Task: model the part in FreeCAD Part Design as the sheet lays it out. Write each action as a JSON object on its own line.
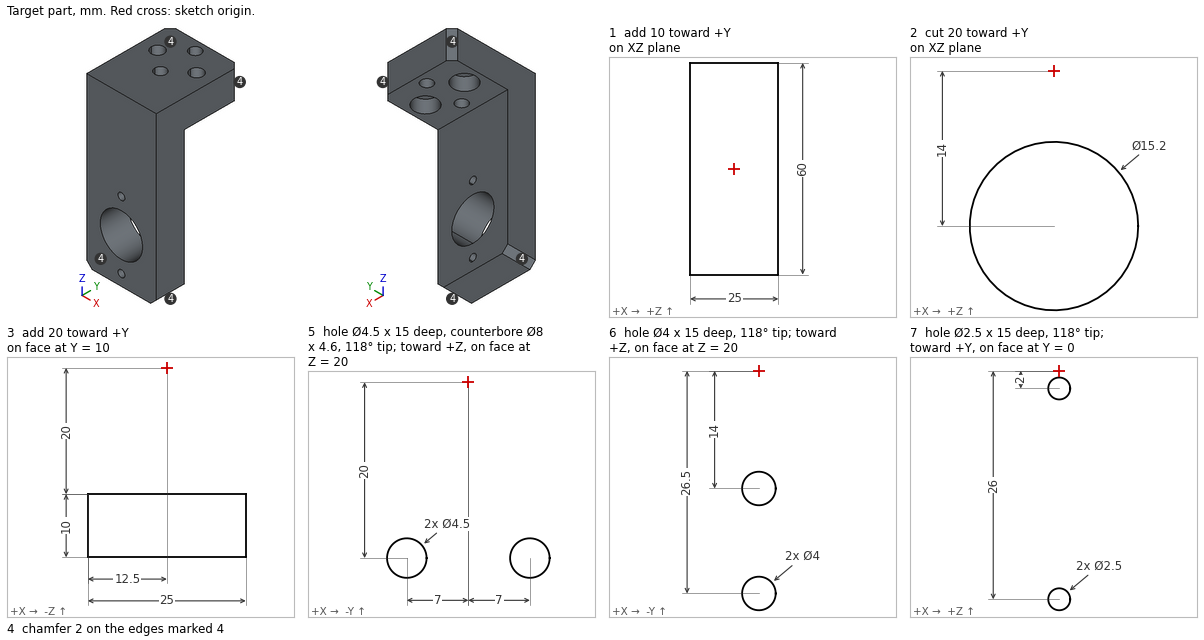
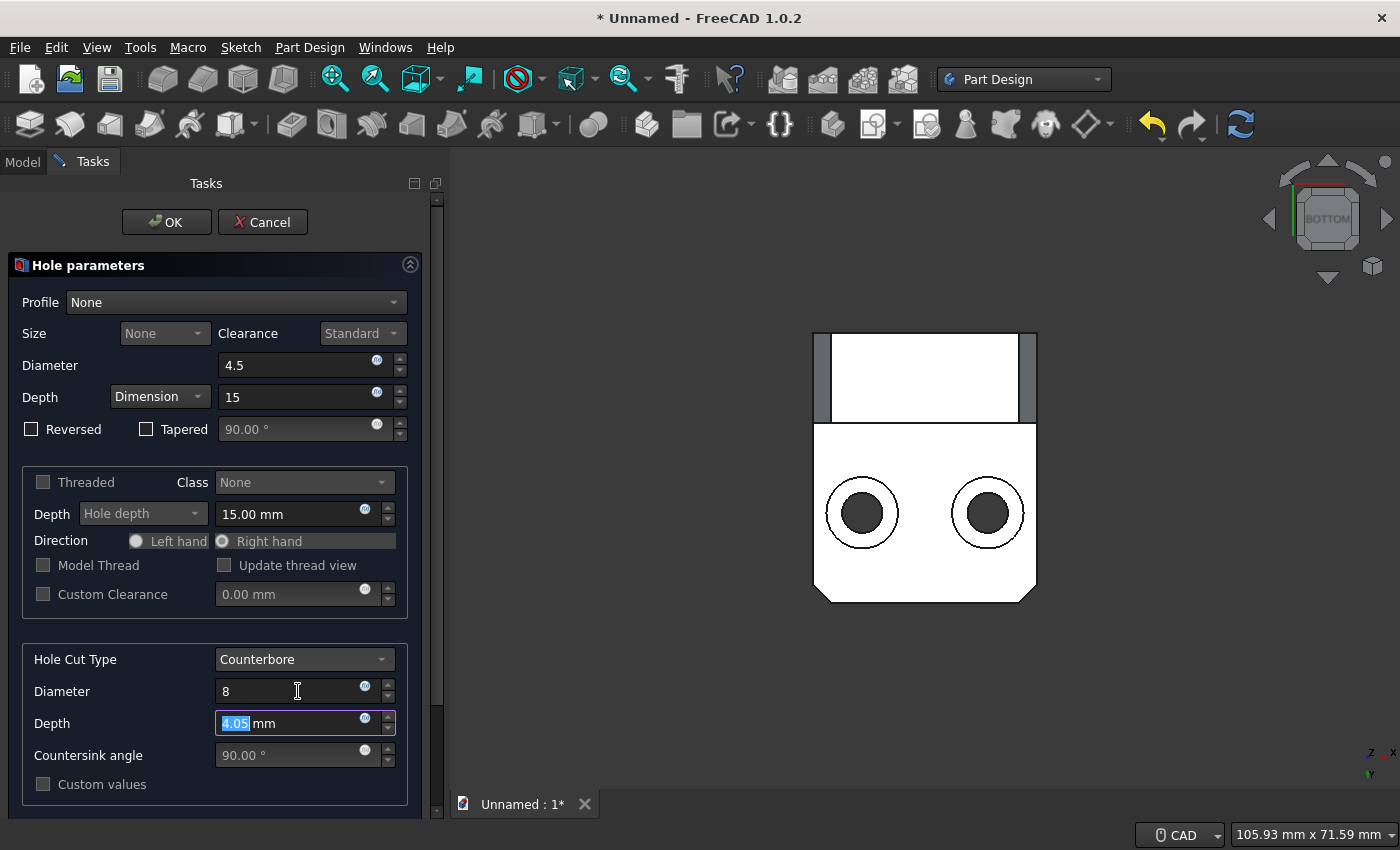
{"action": "type", "text": "4.6"}
{"action": "key", "text": "Tab"}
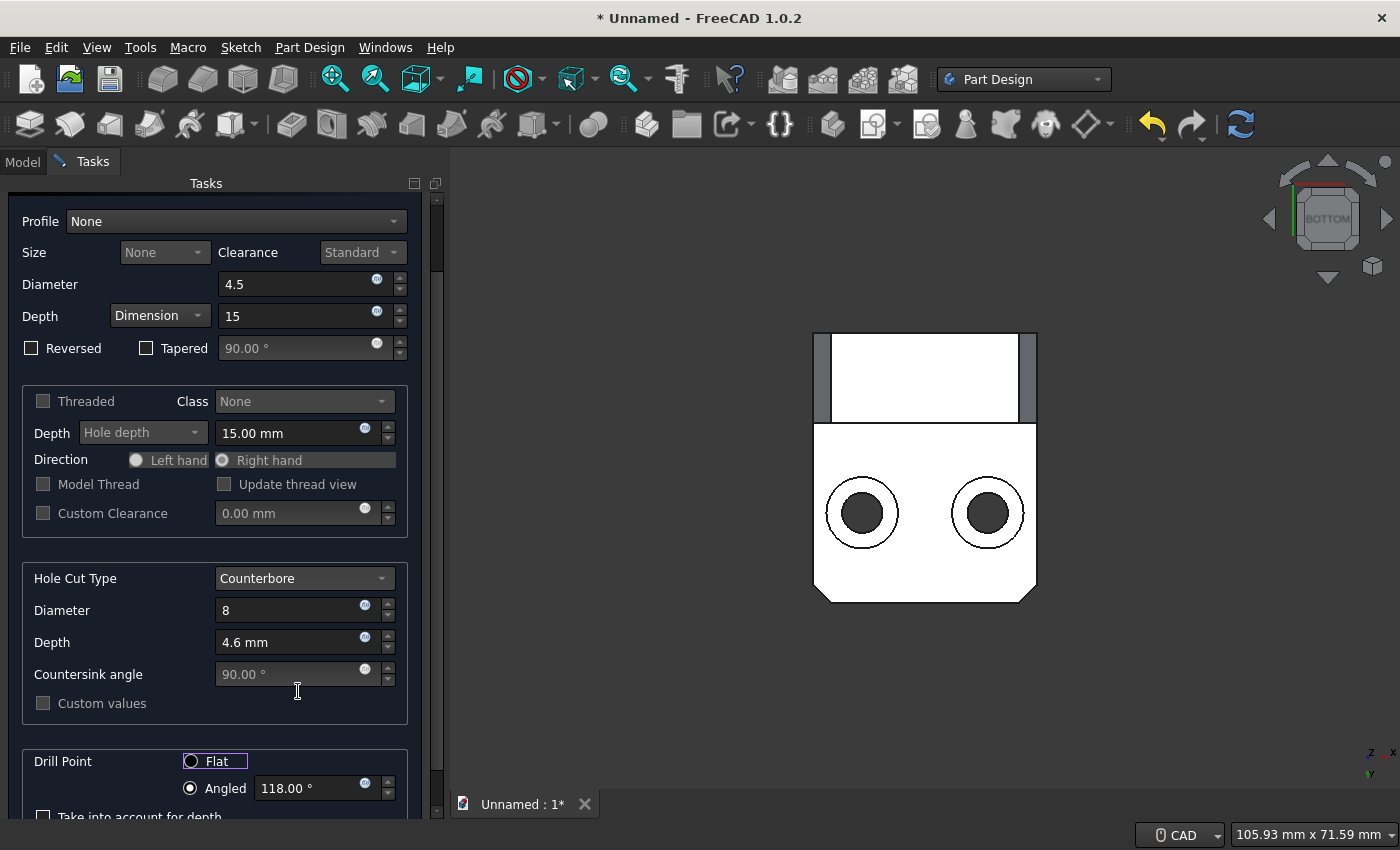
{"action": "scroll", "coordinate": [437, 506], "scroll_direction": "up", "scroll_amount": 3}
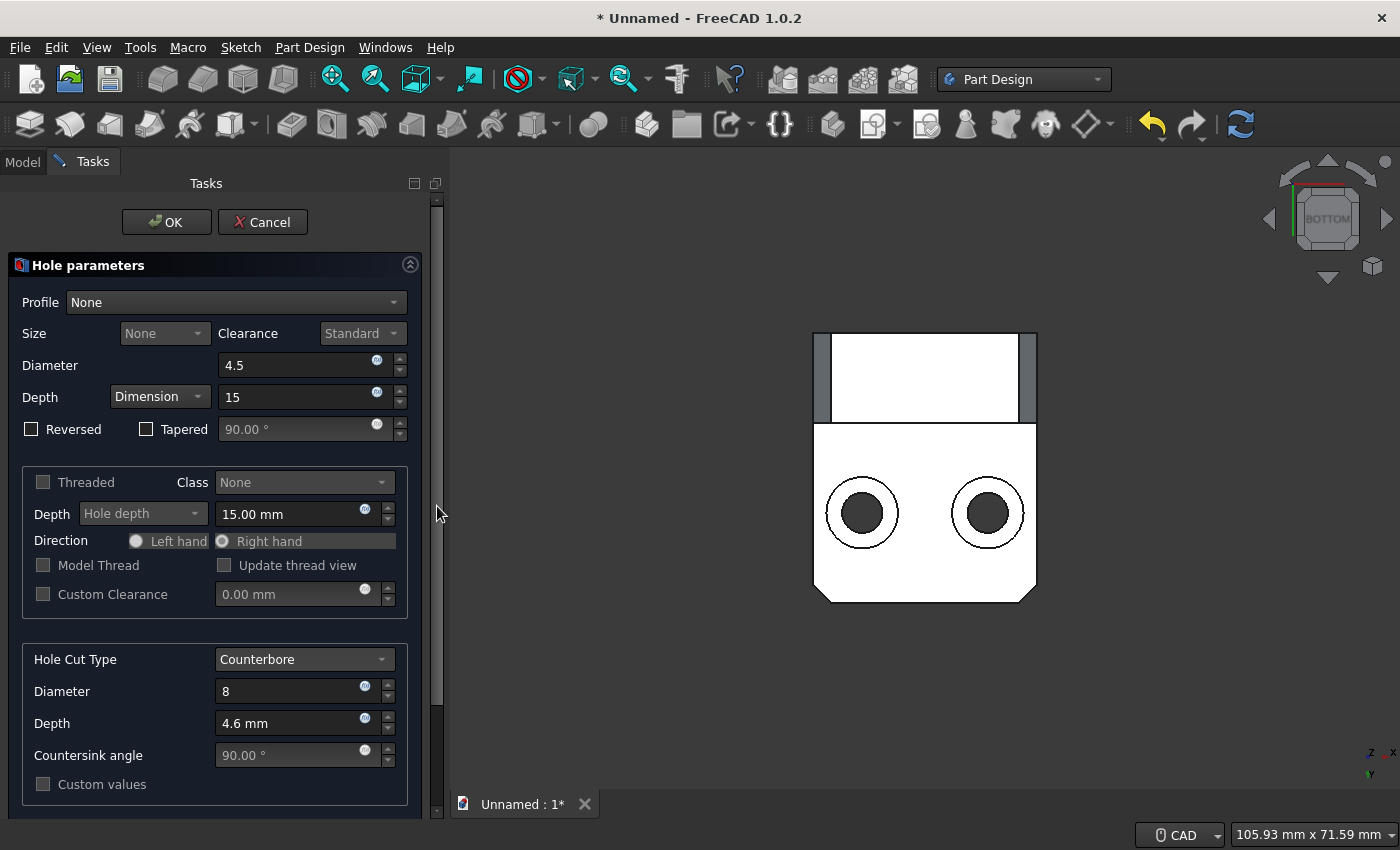
{"action": "left_click", "coordinate": [167, 222]}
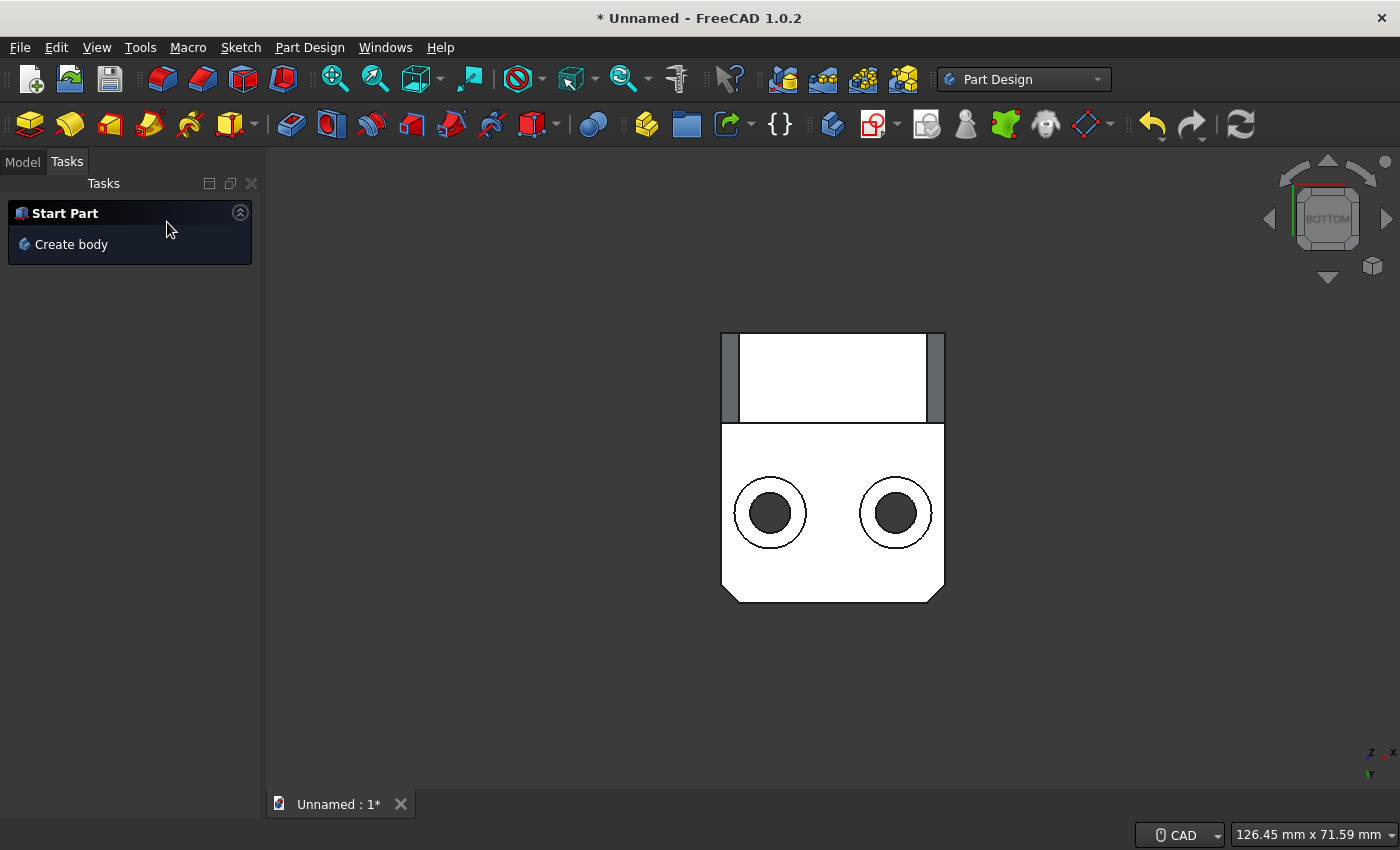
{"action": "key", "text": "v f"}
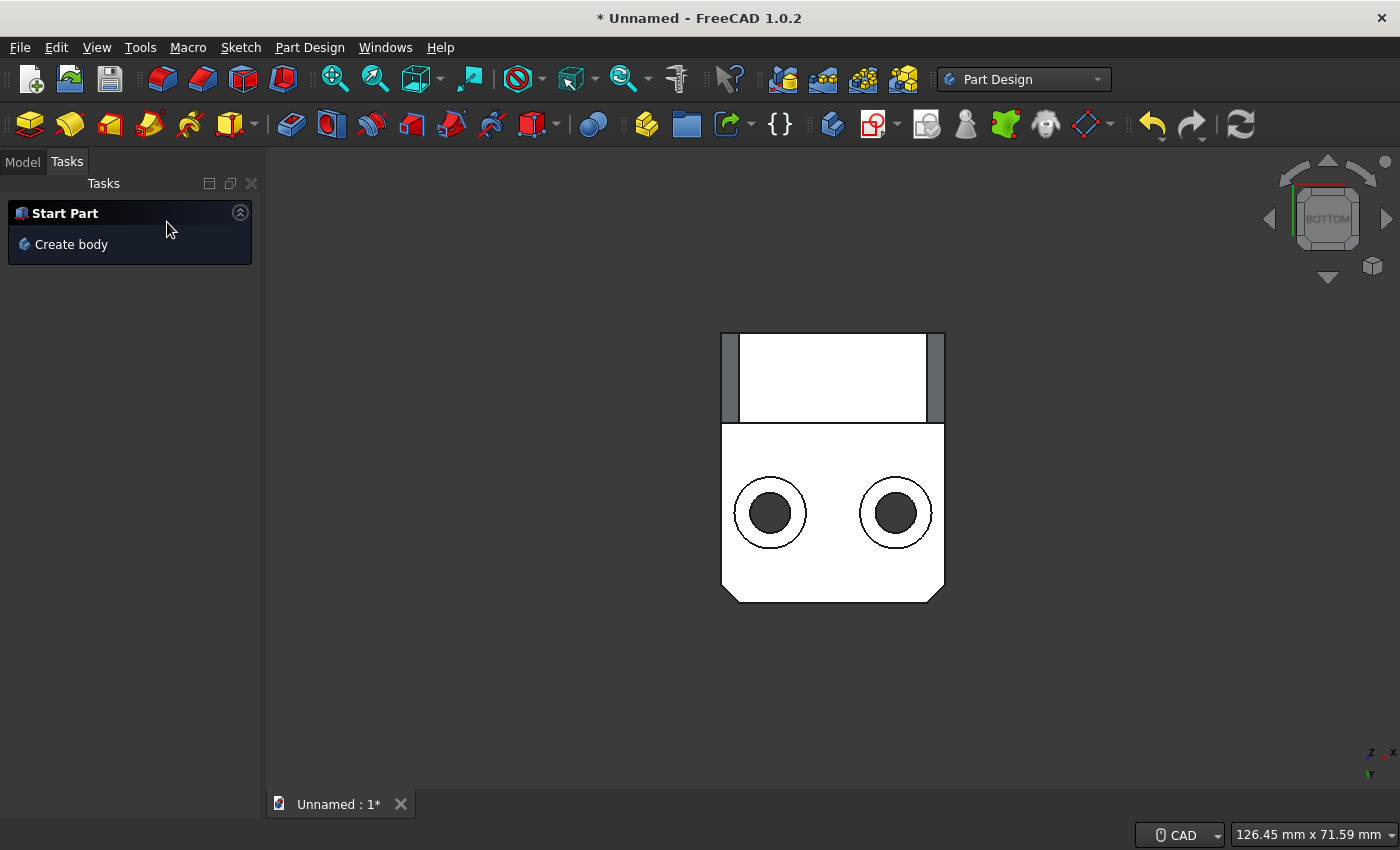
{"action": "left_click", "coordinate": [833, 461]}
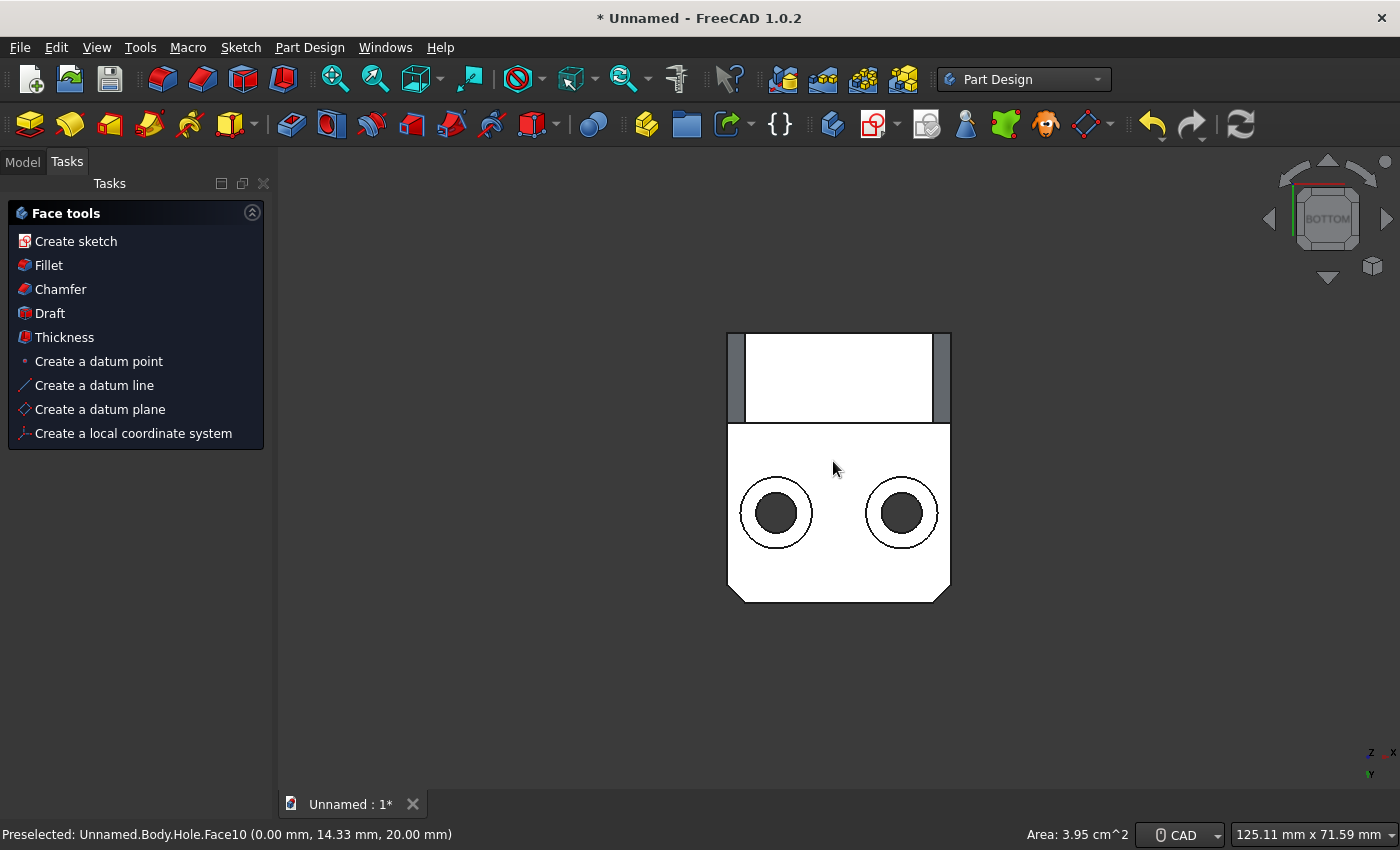
{"action": "left_click", "coordinate": [874, 124]}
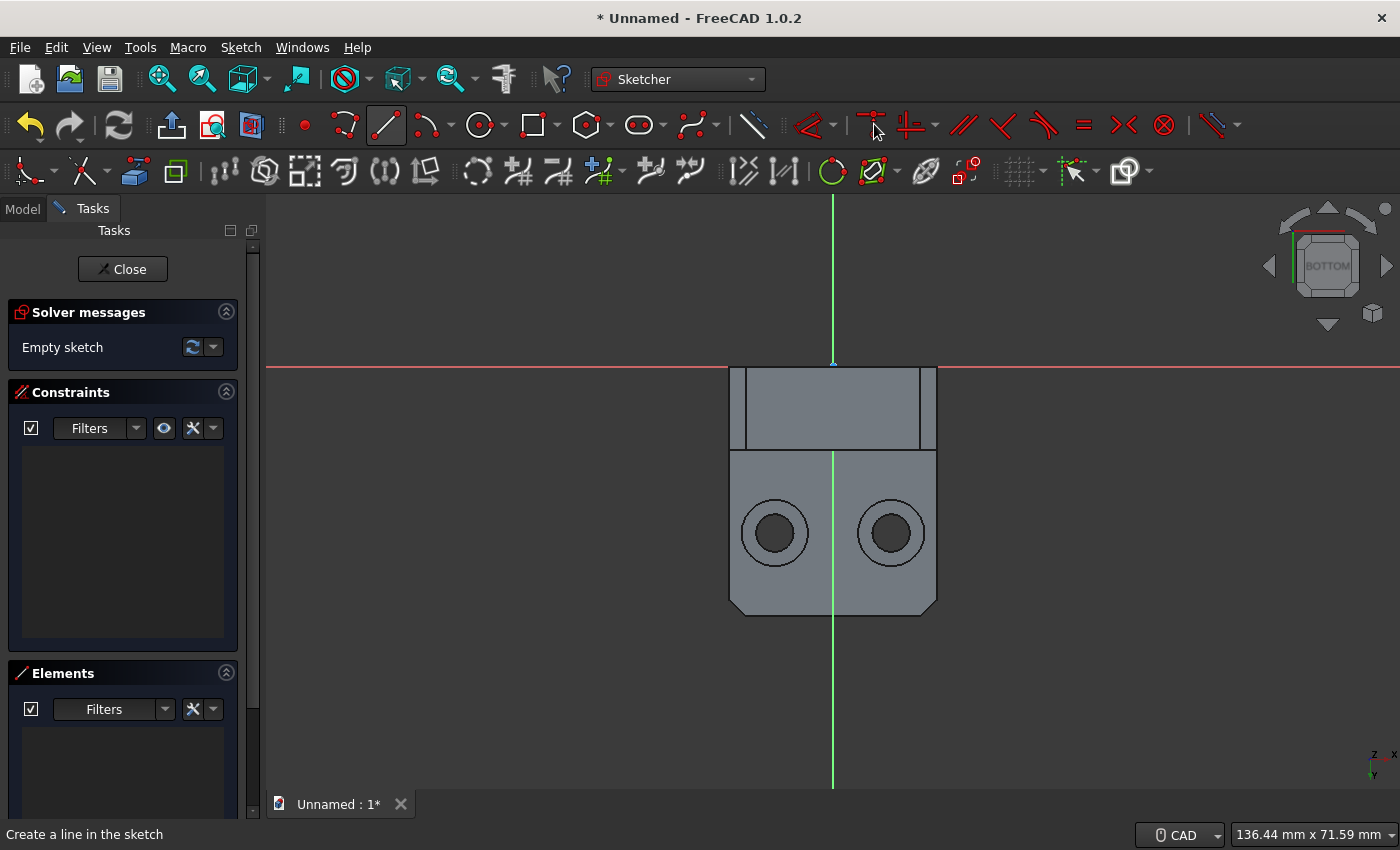
{"action": "scroll", "coordinate": [972, 473], "scroll_direction": "up", "scroll_amount": 2}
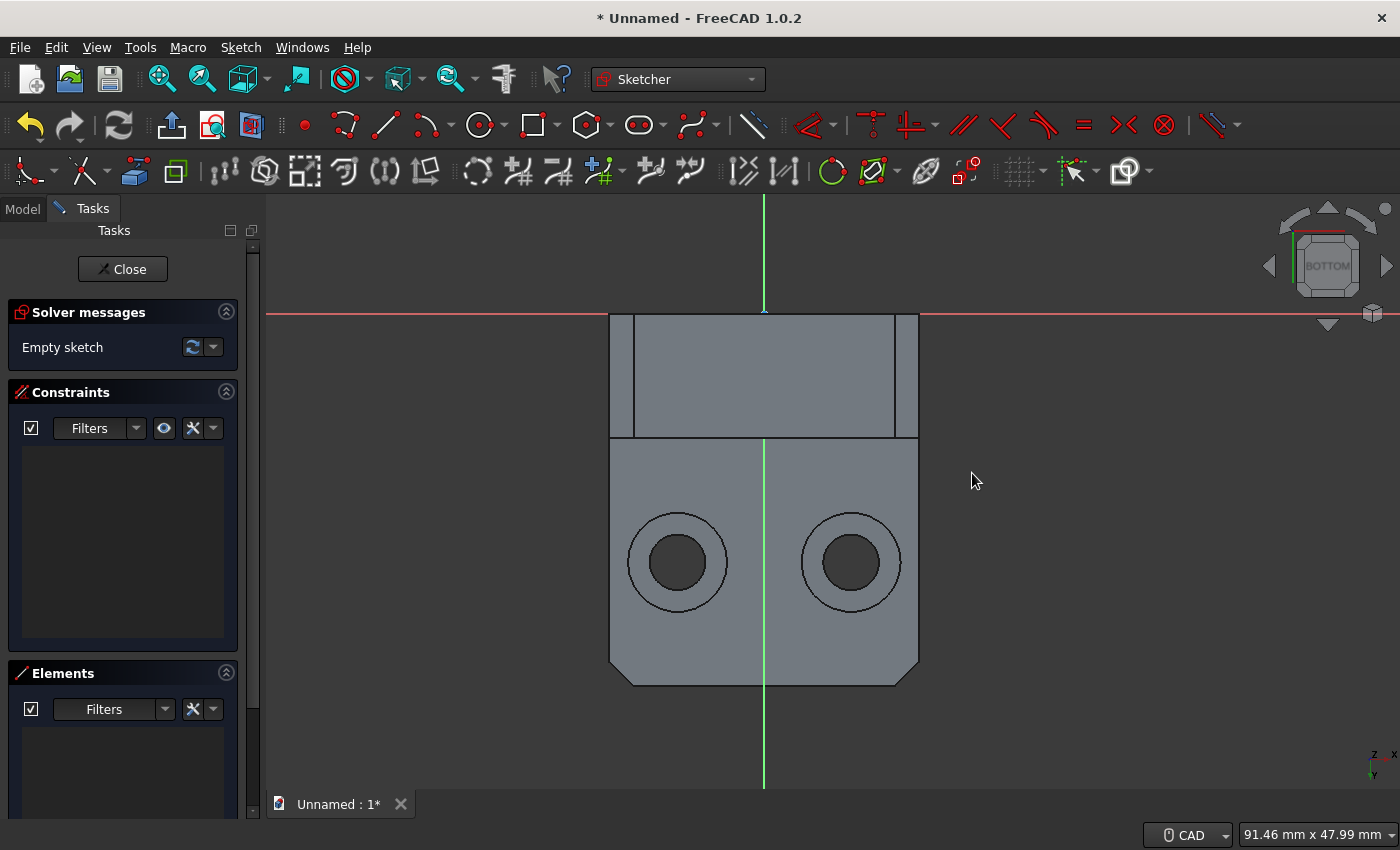
{"action": "key", "text": "g c"}